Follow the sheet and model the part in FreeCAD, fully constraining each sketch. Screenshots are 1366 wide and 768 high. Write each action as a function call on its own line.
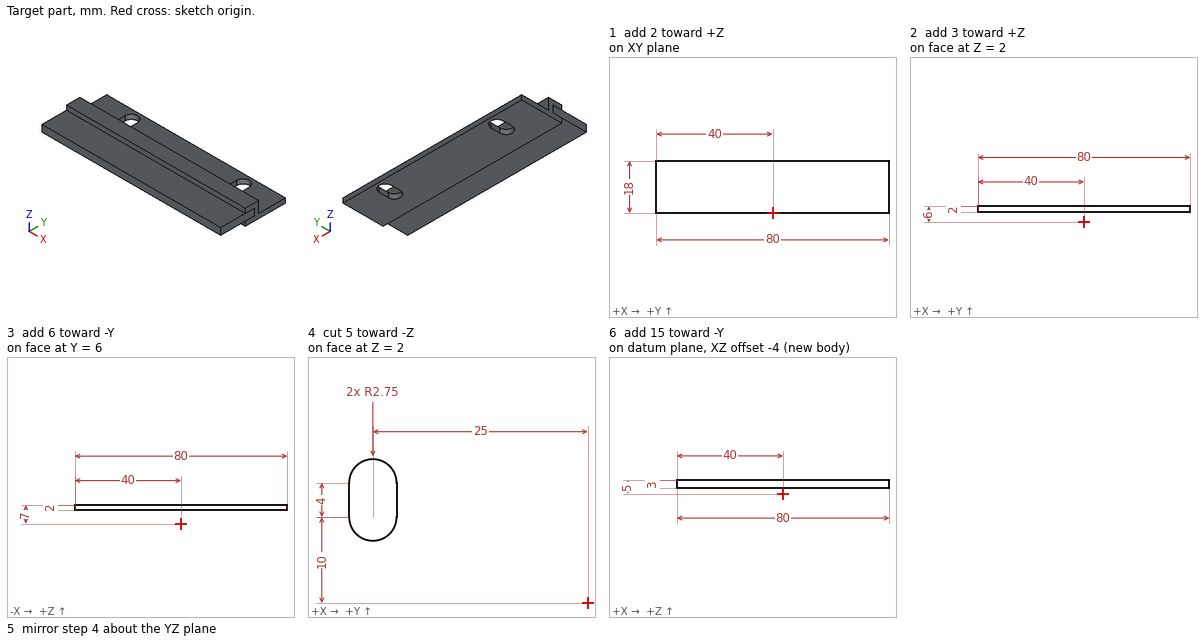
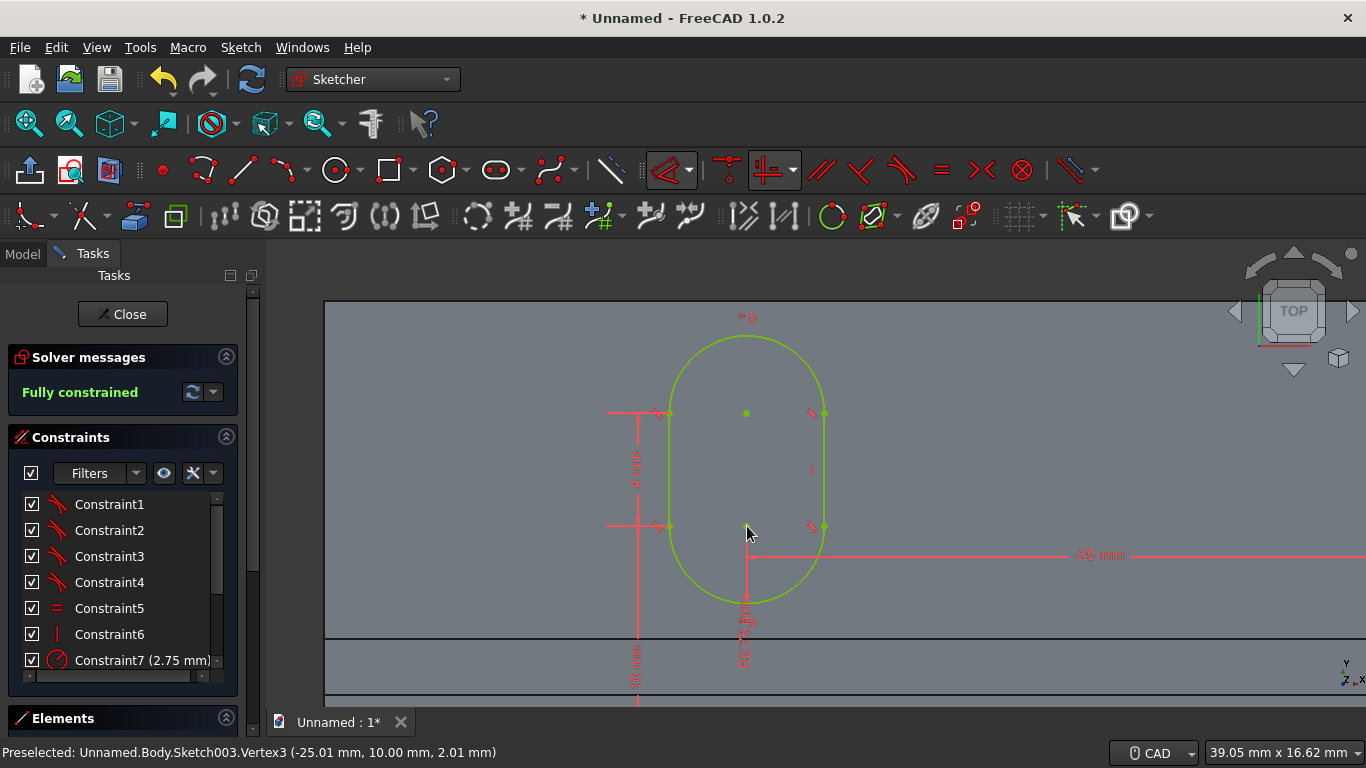
click(123, 314)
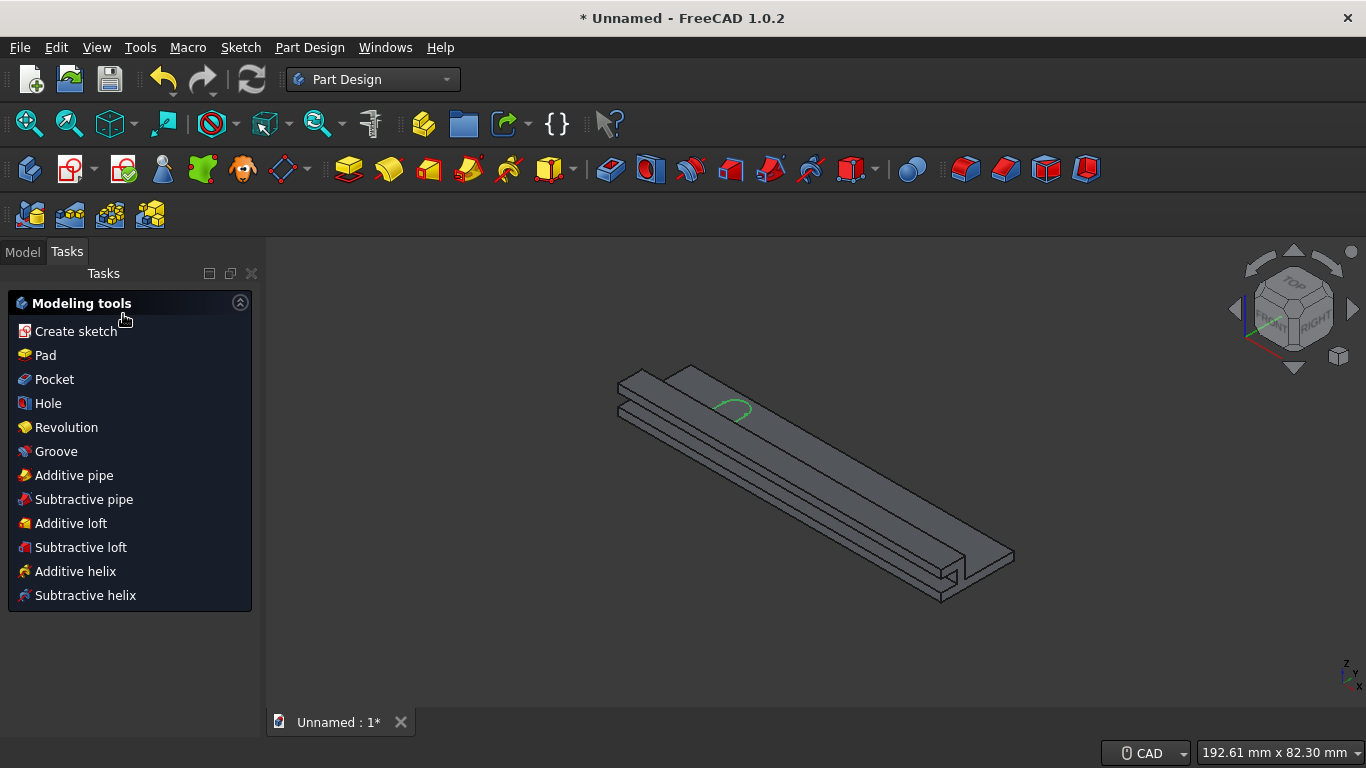
click(612, 170)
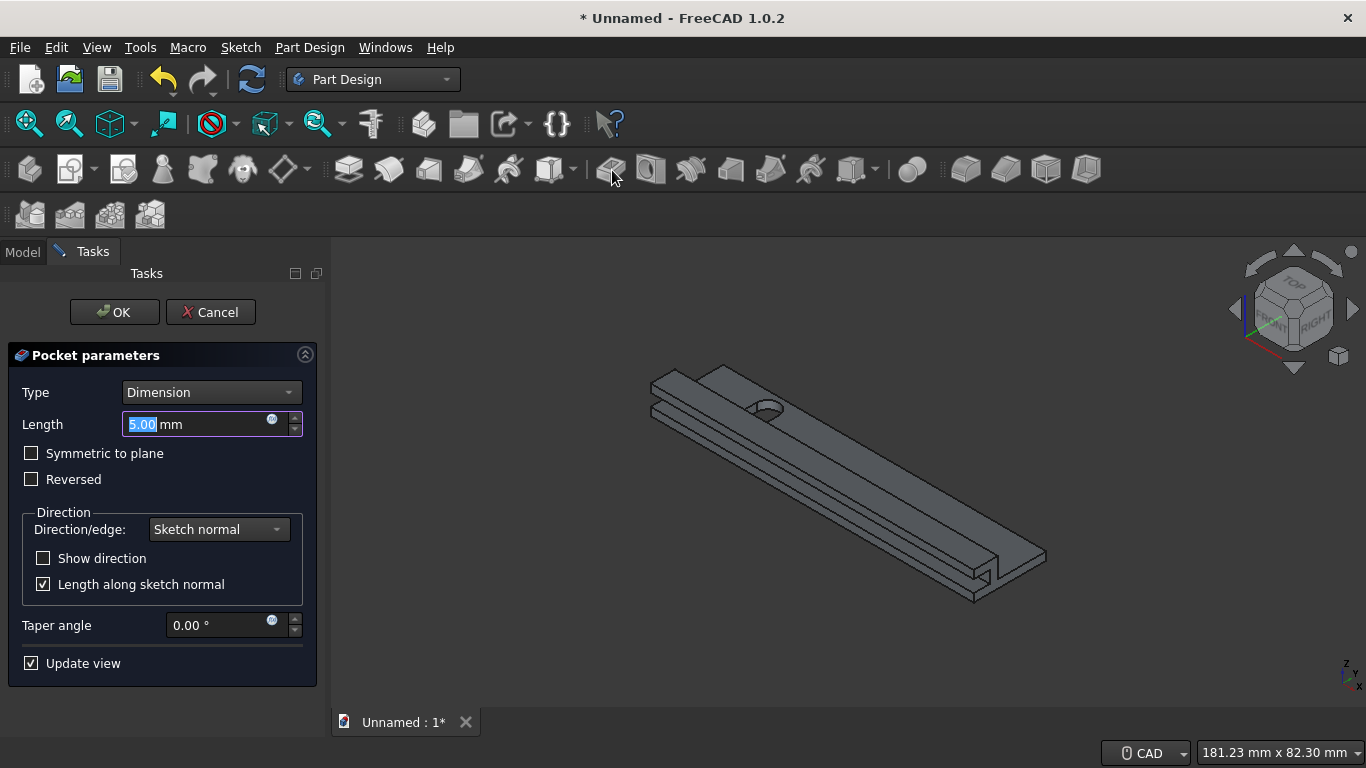
text(5)
key(Tab)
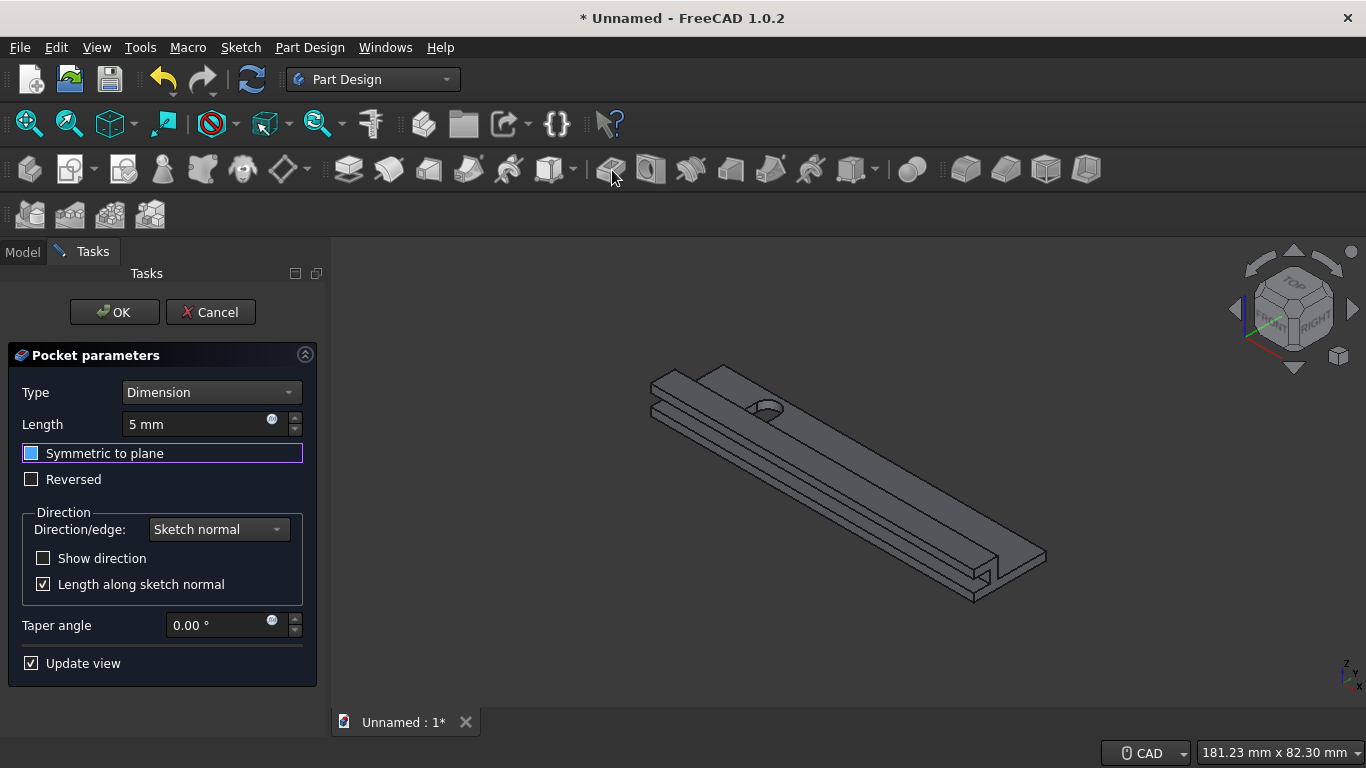
click(115, 312)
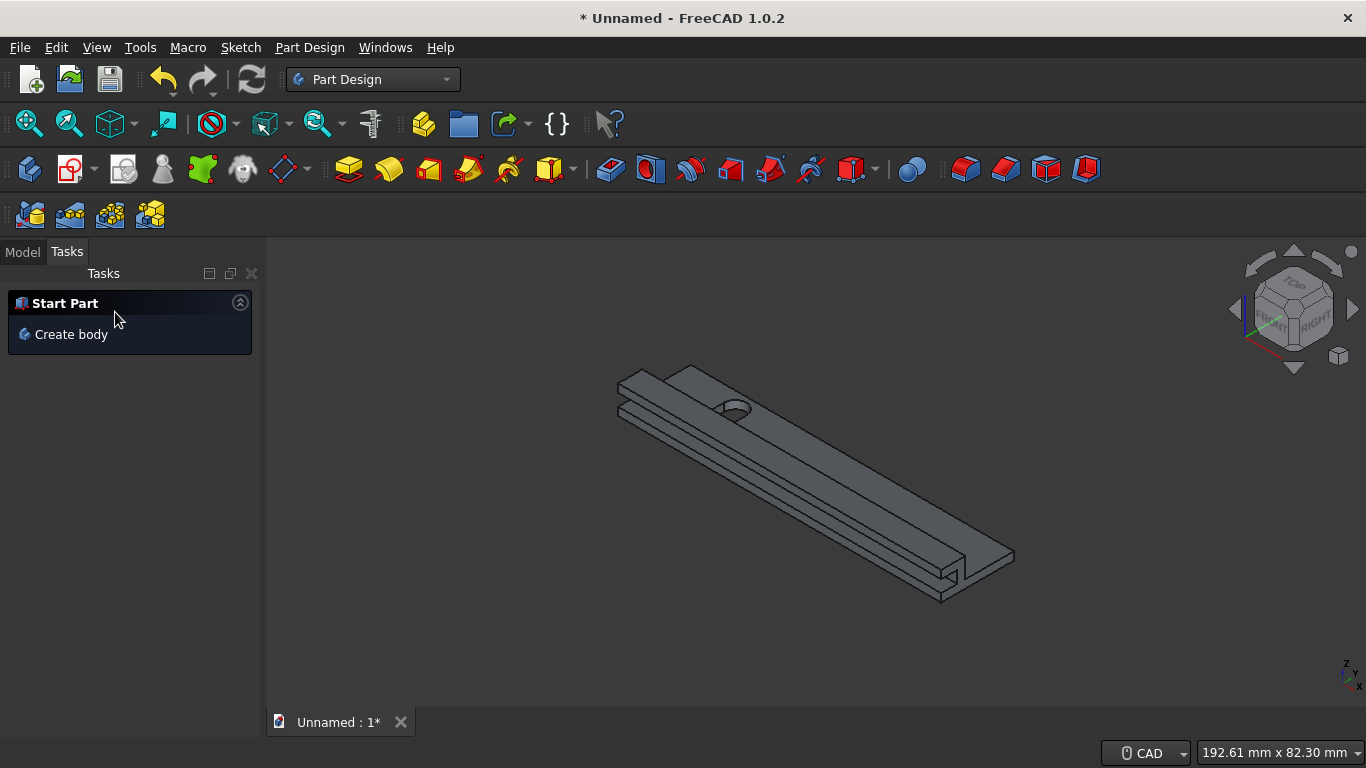
click(23, 251)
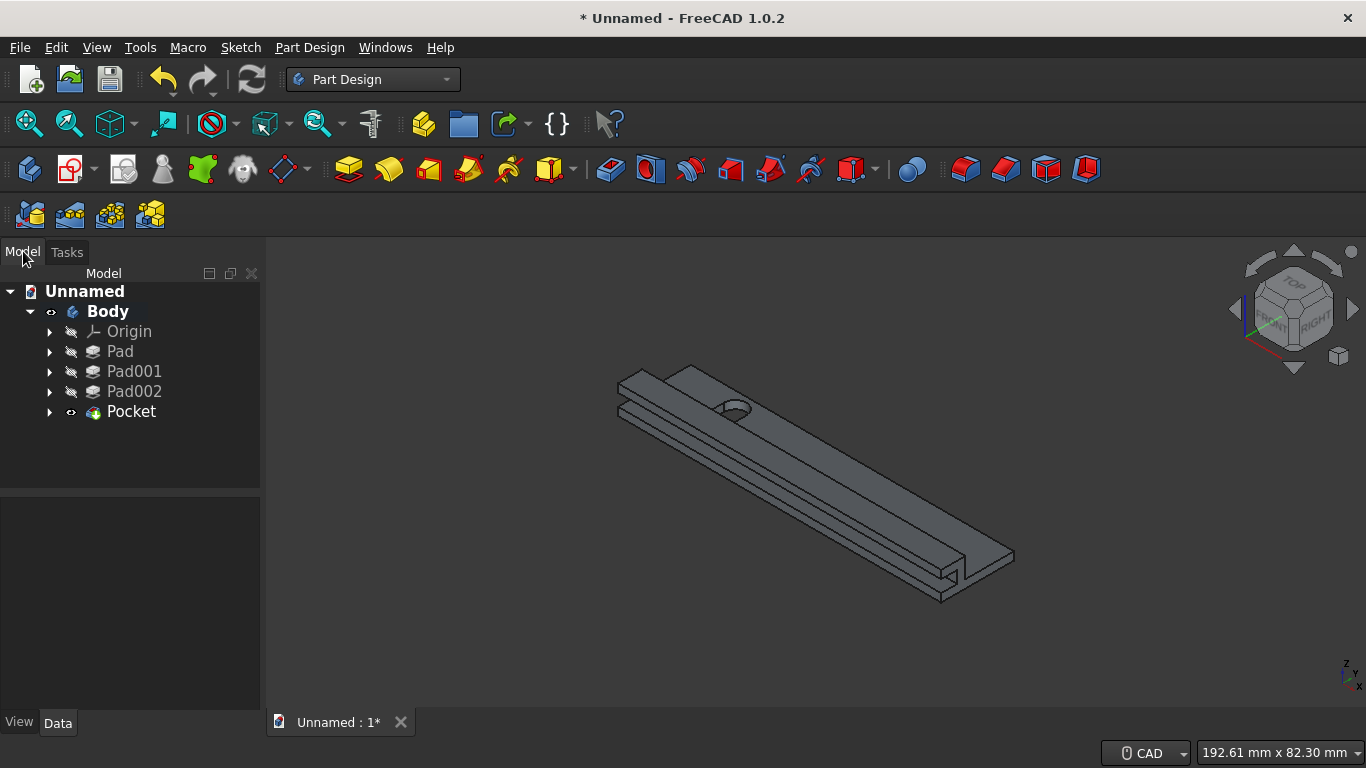
click(116, 412)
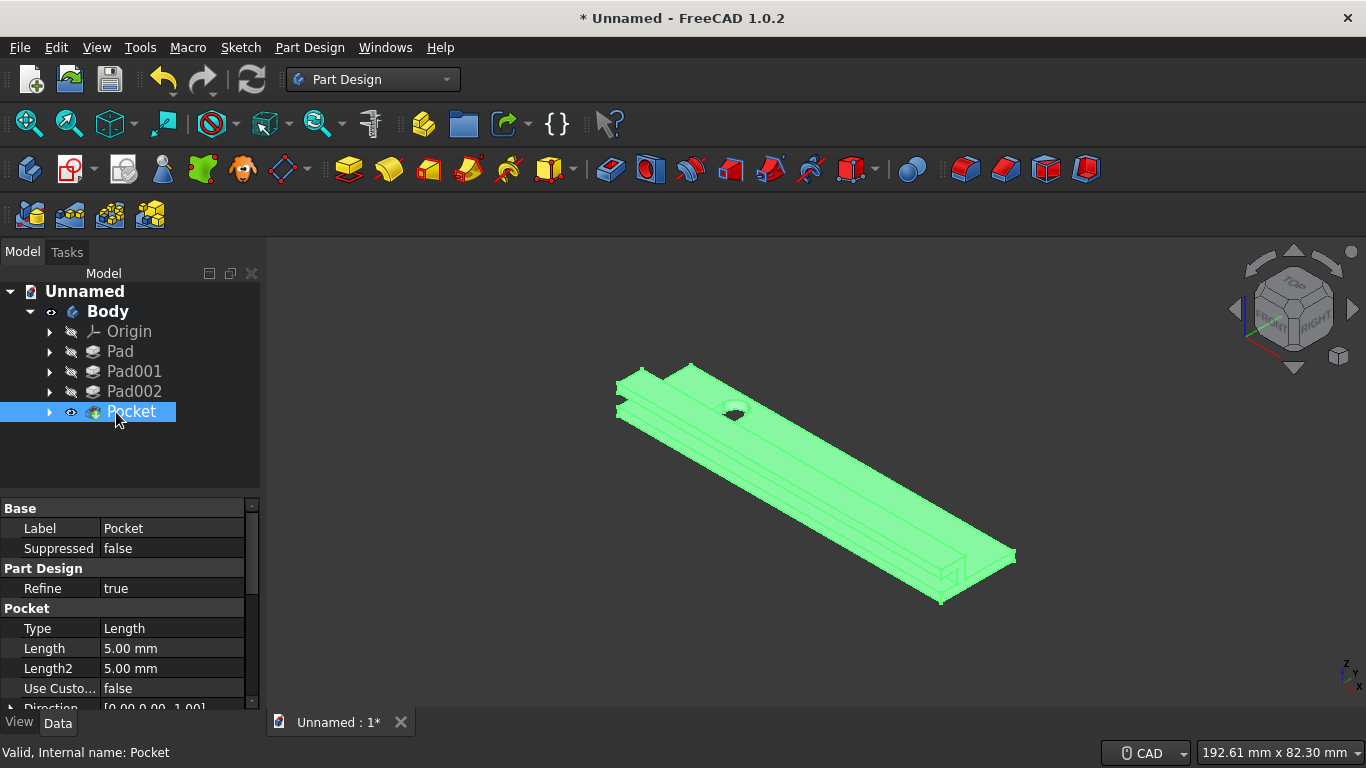
click(30, 214)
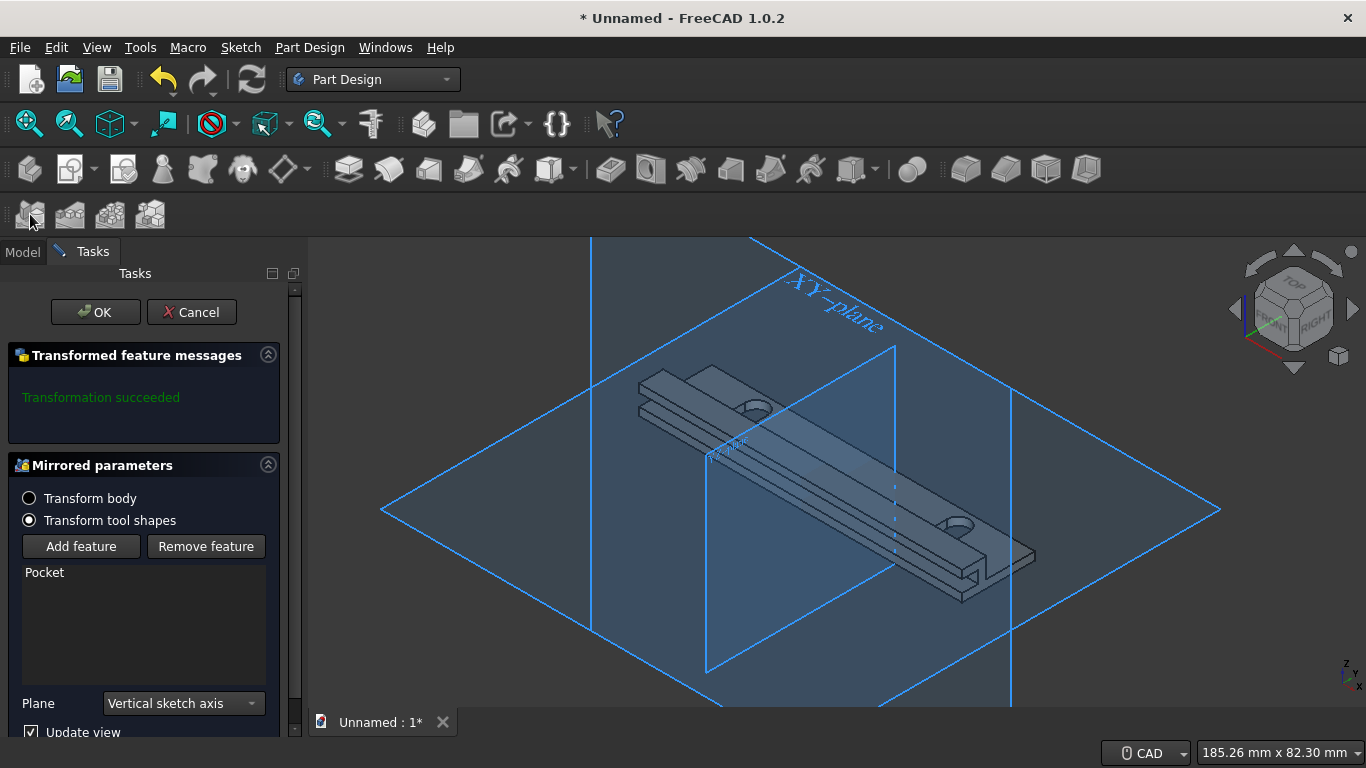
click(184, 704)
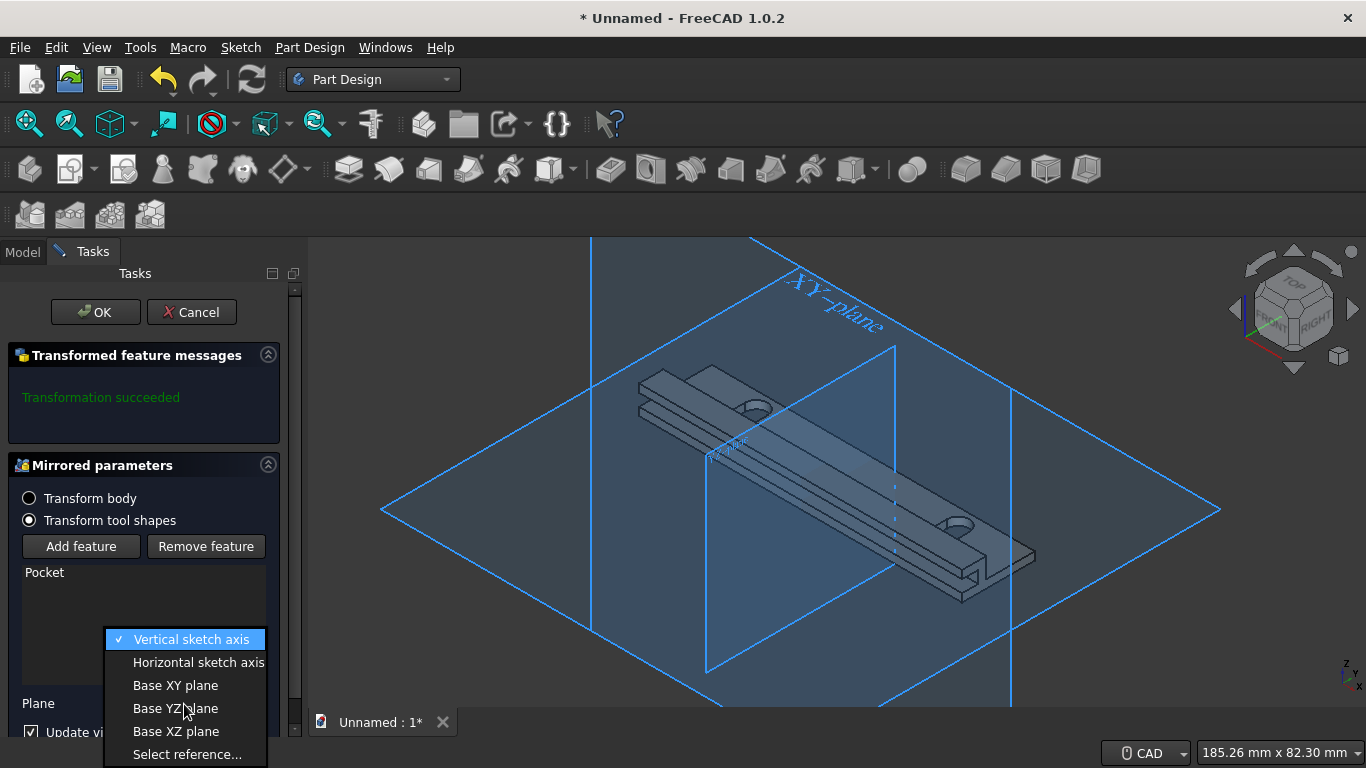
click(184, 708)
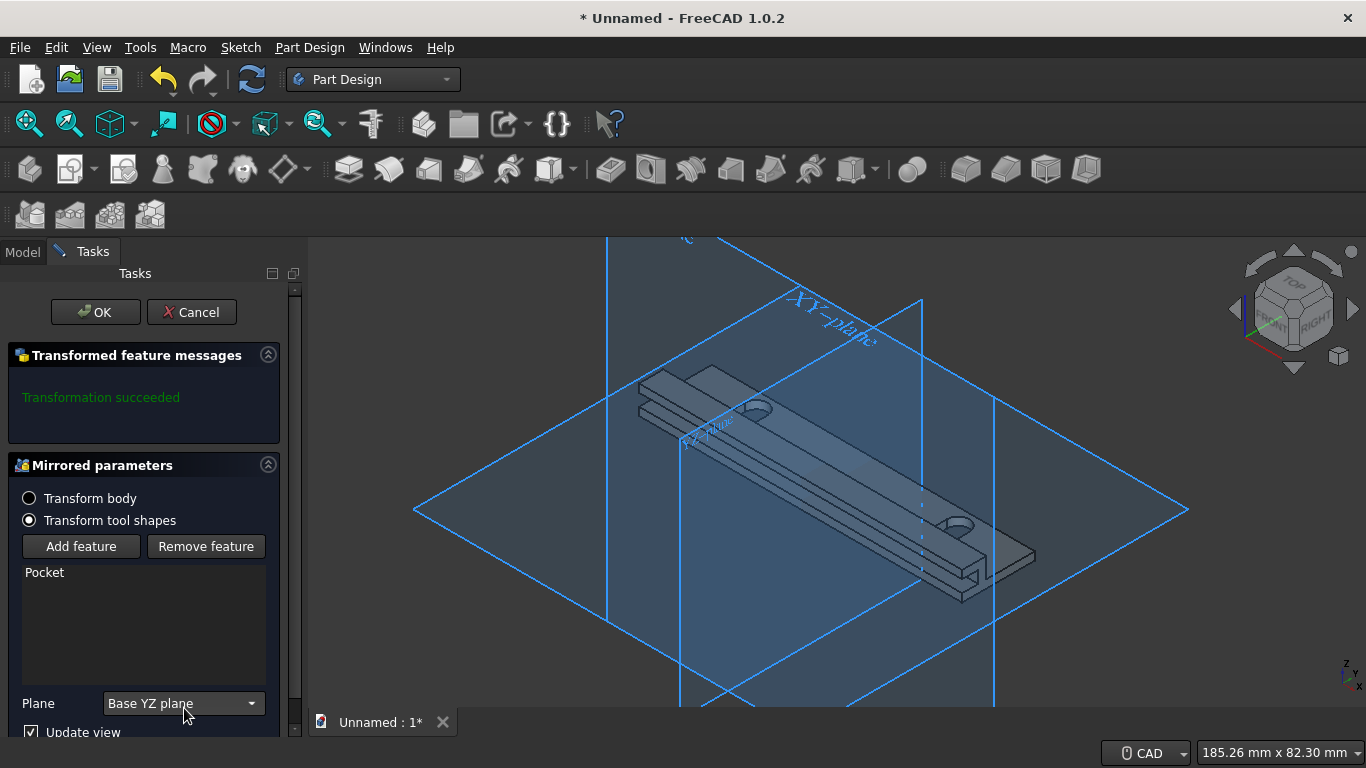
click(96, 312)